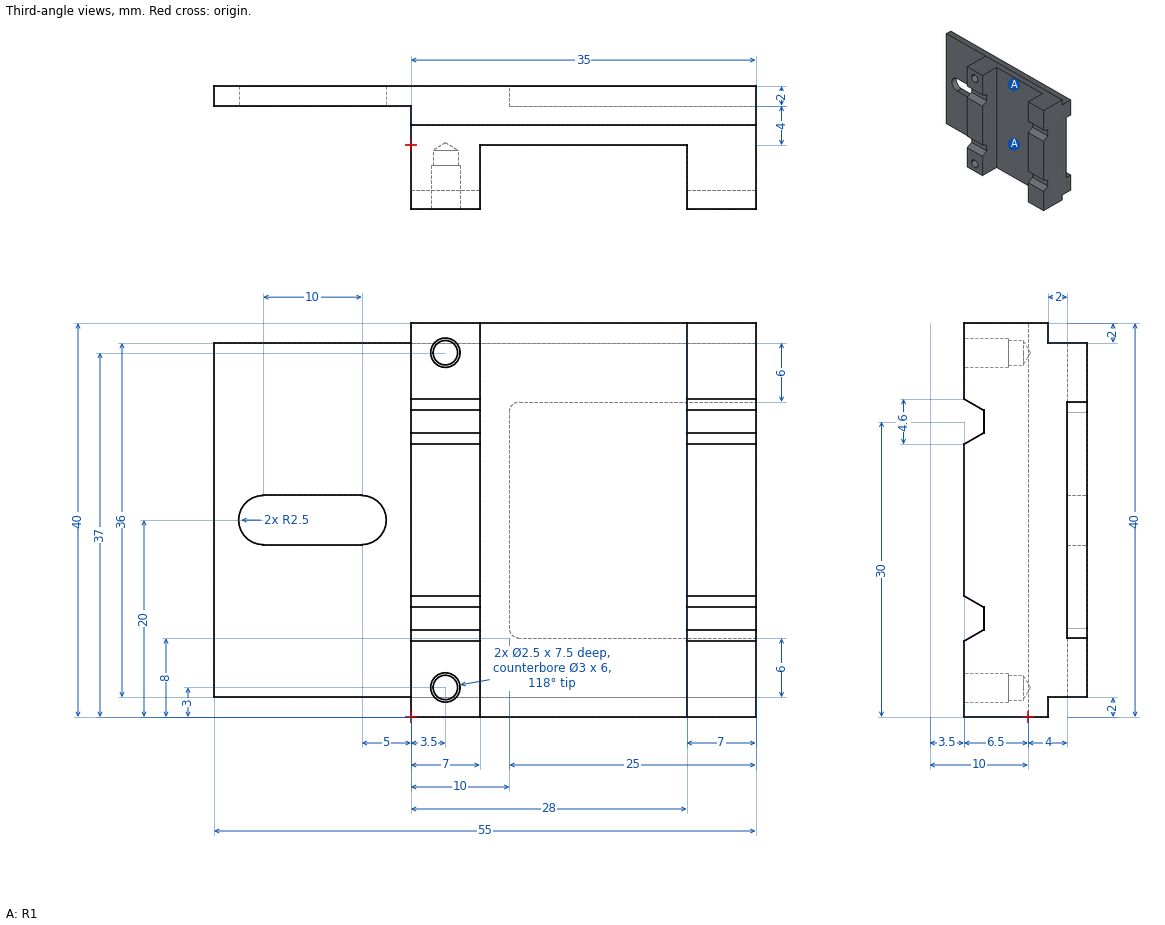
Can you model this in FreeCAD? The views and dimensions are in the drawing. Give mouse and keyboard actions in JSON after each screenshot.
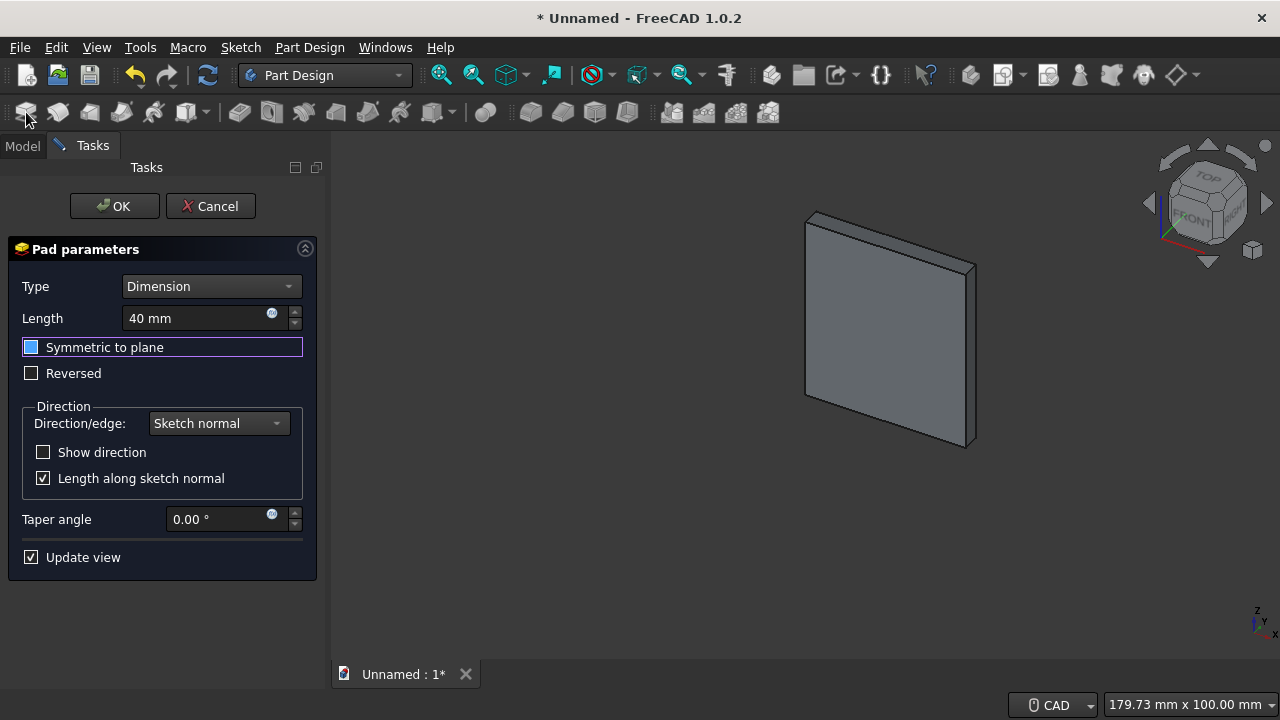
{"action": "left_click", "coordinate": [115, 206]}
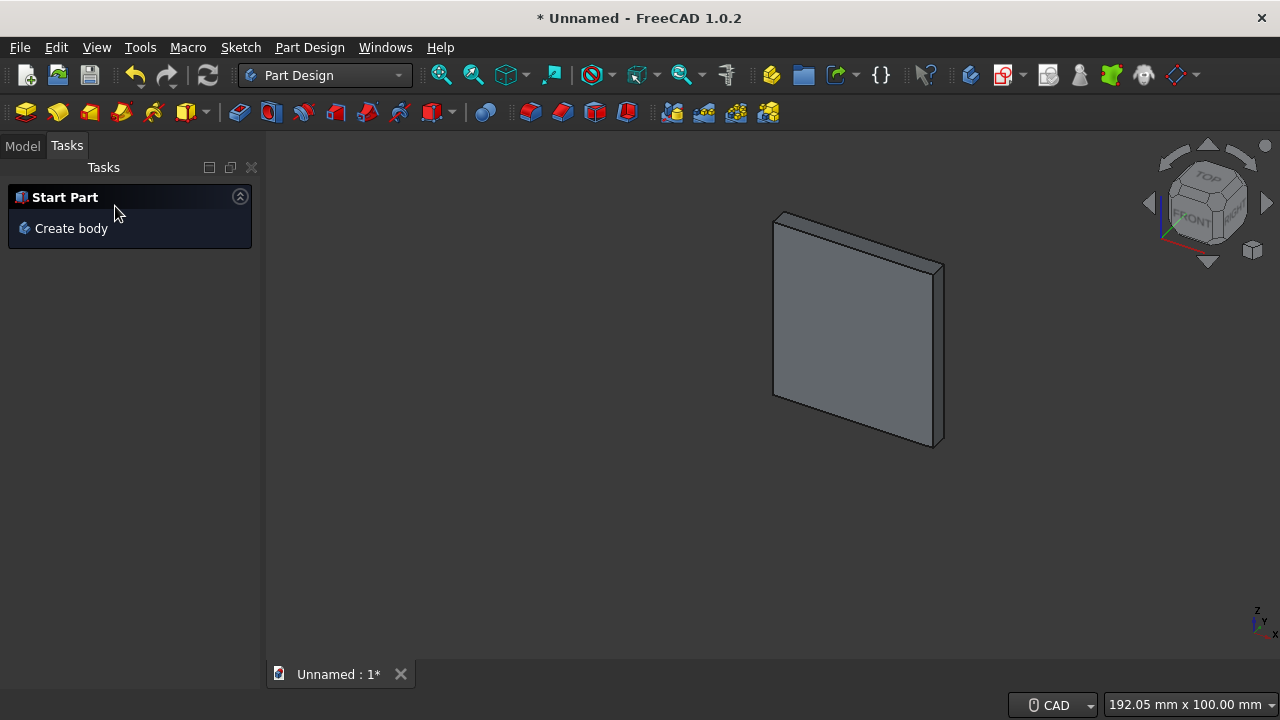
{"action": "left_click", "coordinate": [442, 76]}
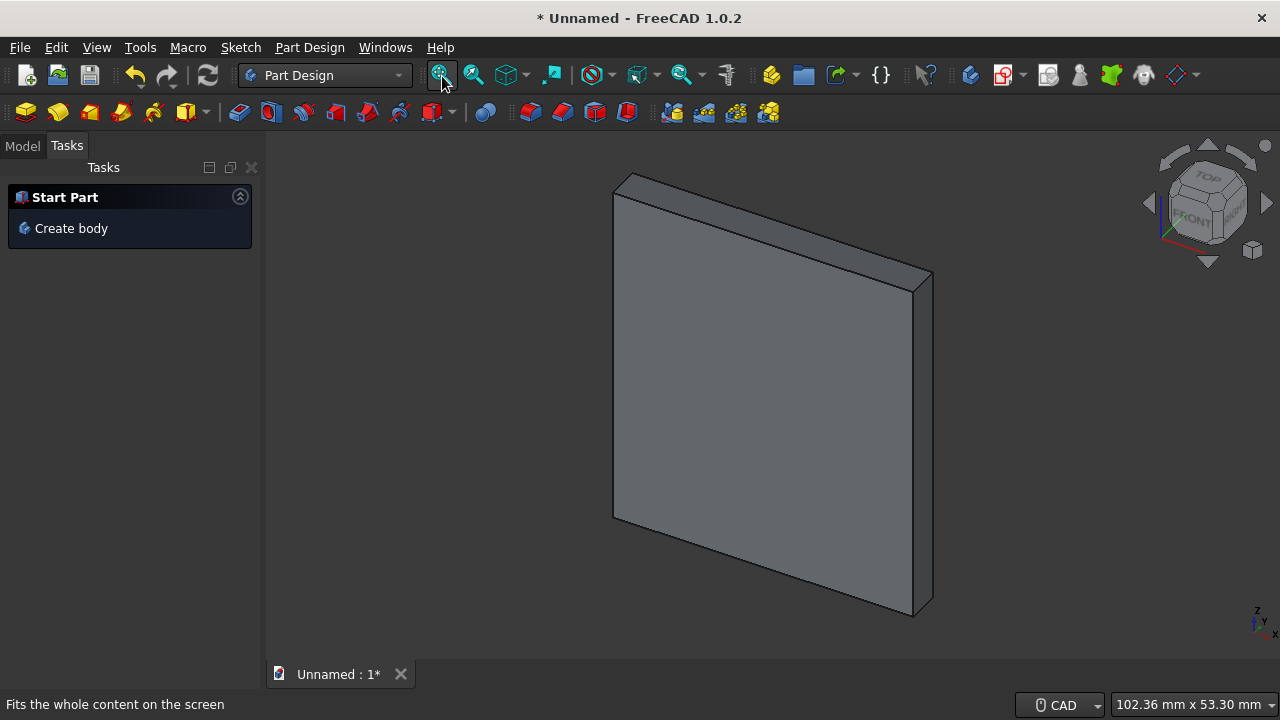
{"action": "key", "text": "4"}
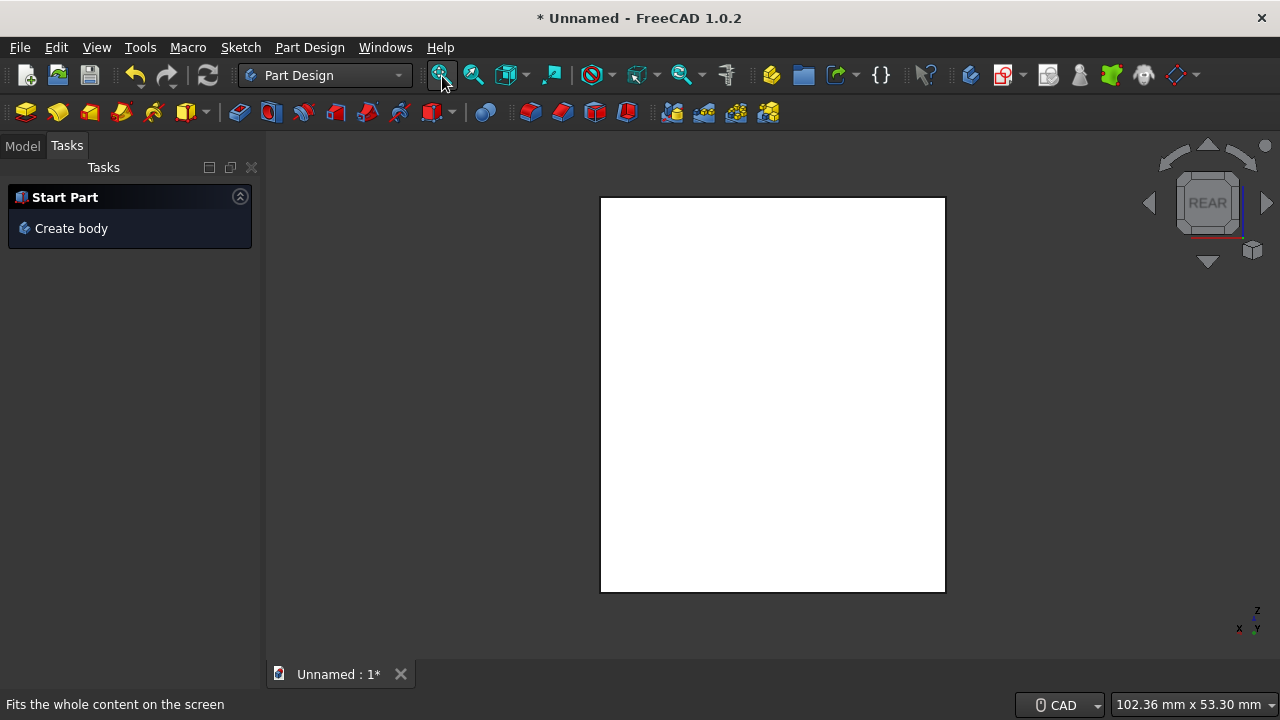
{"action": "left_click", "coordinate": [773, 394]}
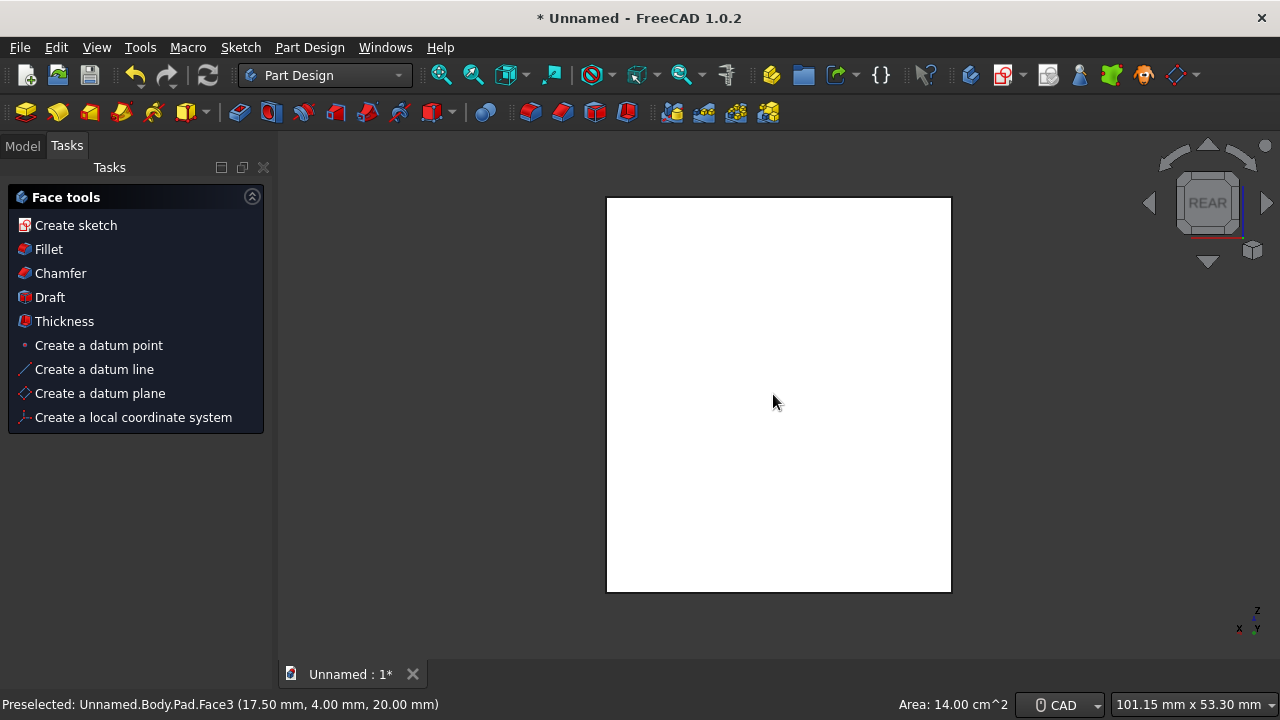
{"action": "left_click", "coordinate": [1004, 76]}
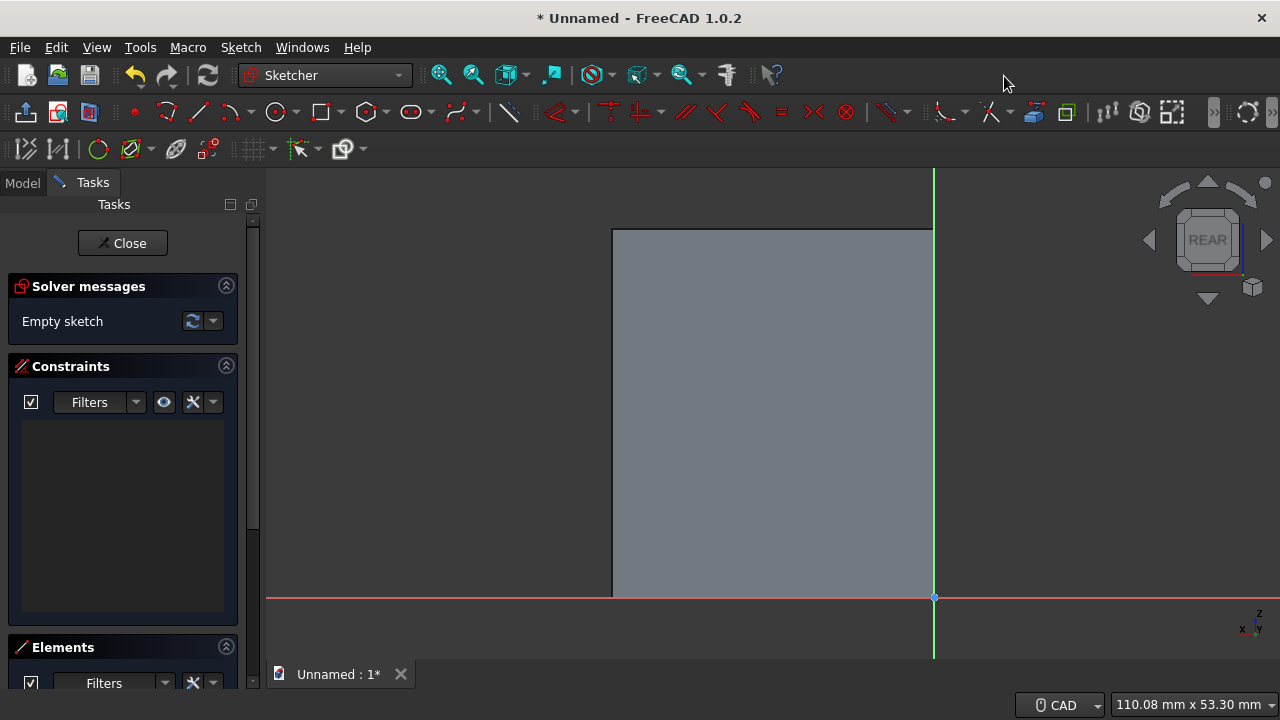
{"action": "left_click", "coordinate": [322, 112]}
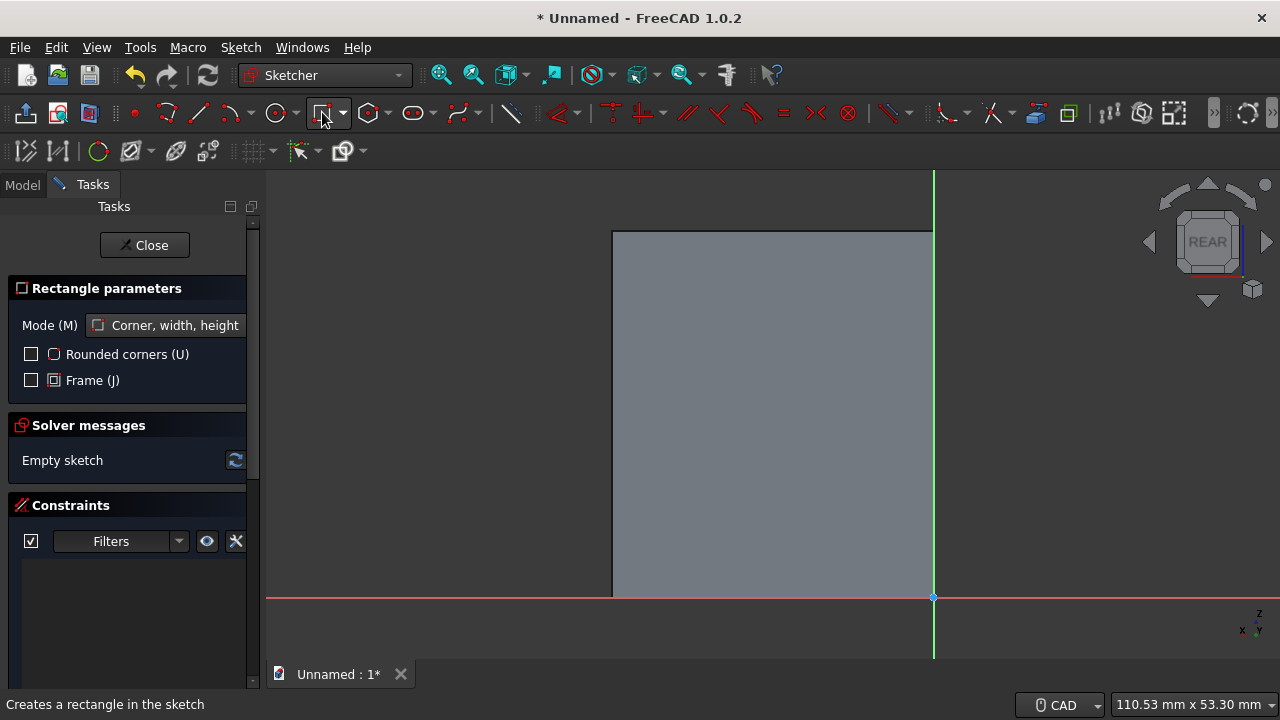
{"action": "left_click", "coordinate": [934, 598]}
{"action": "mouse_move", "coordinate": [869, 231]}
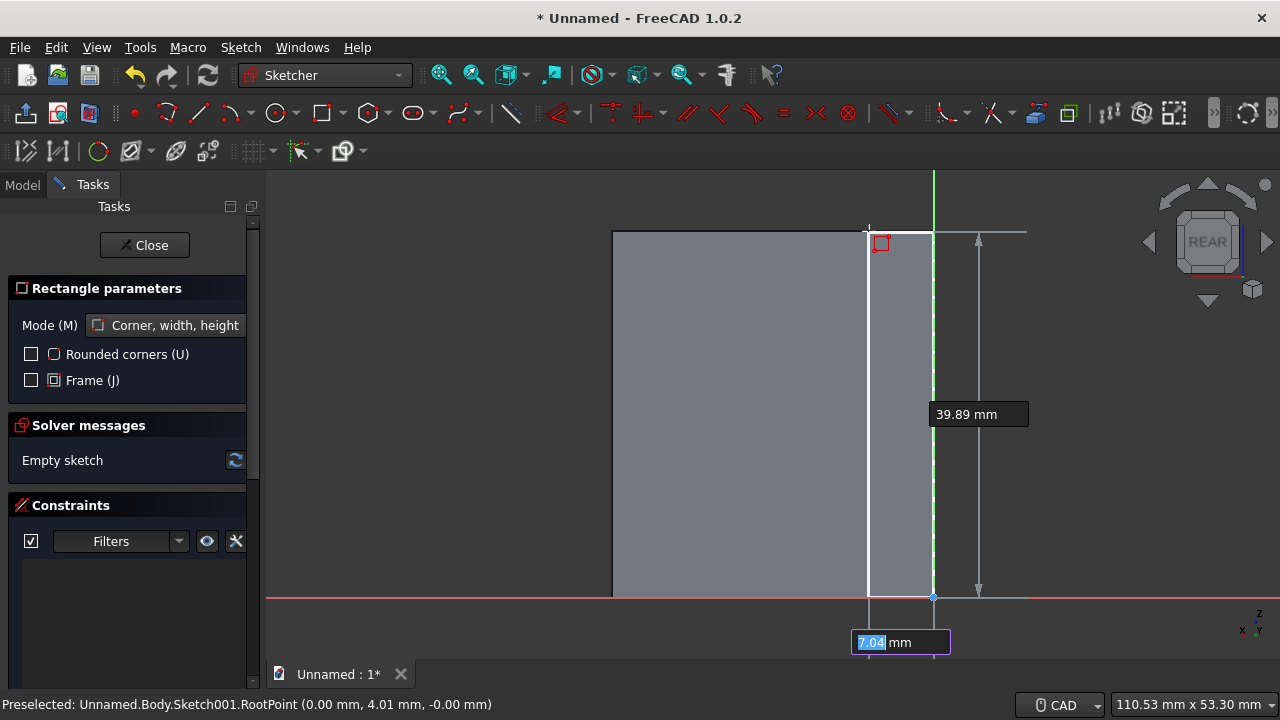
{"action": "type", "text": "7"}
{"action": "key", "text": "Tab"}
{"action": "type", "text": "40"}
{"action": "key", "text": "Return"}
{"action": "key", "text": "Escape"}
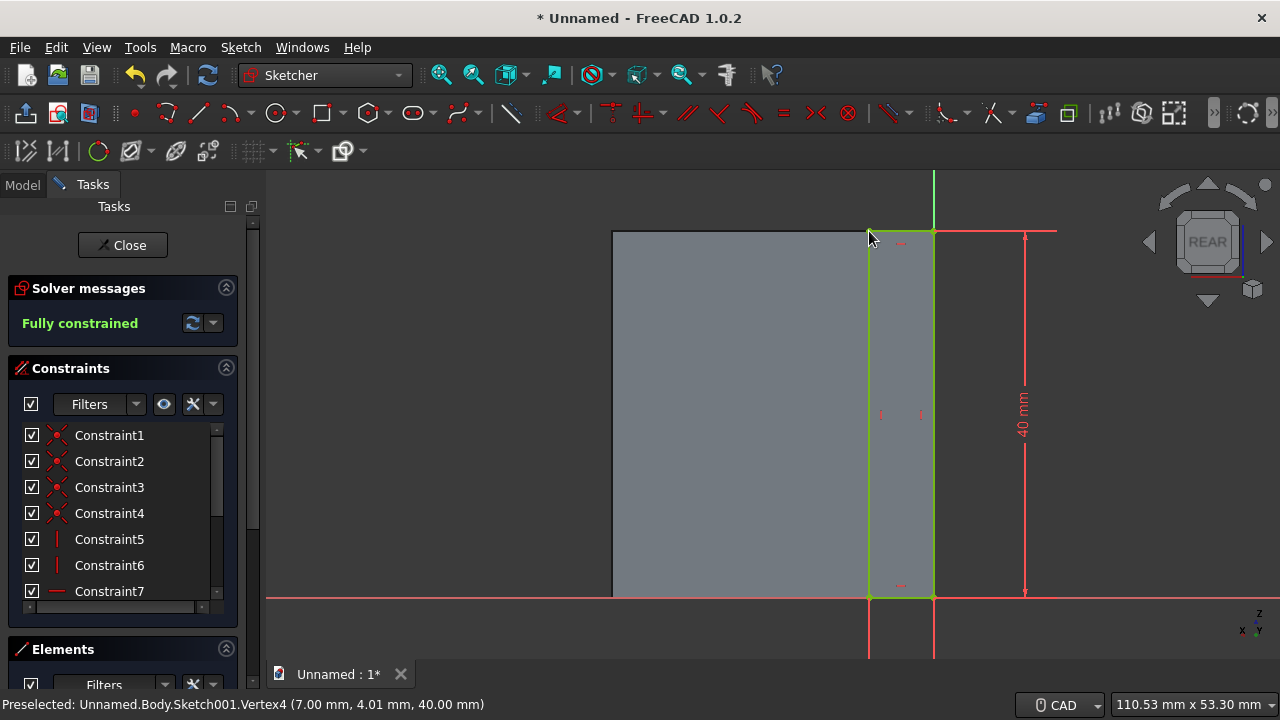
{"action": "left_click", "coordinate": [123, 245]}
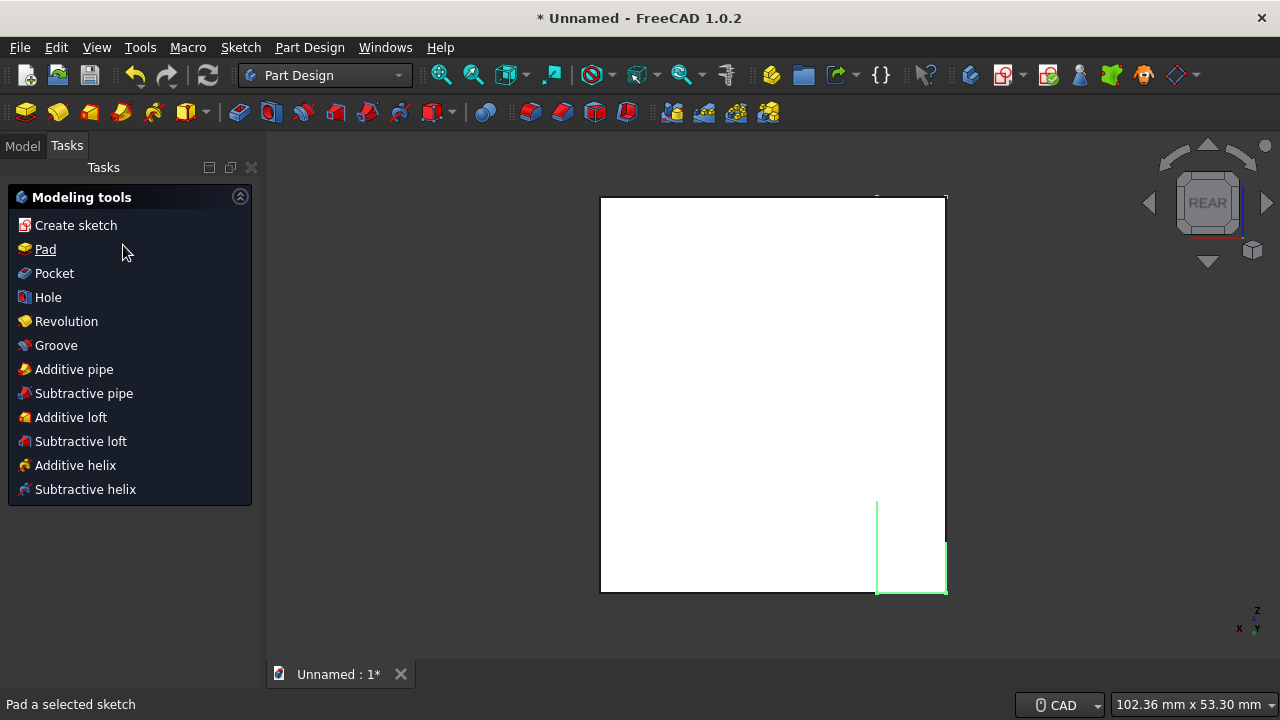
{"action": "left_click", "coordinate": [26, 112]}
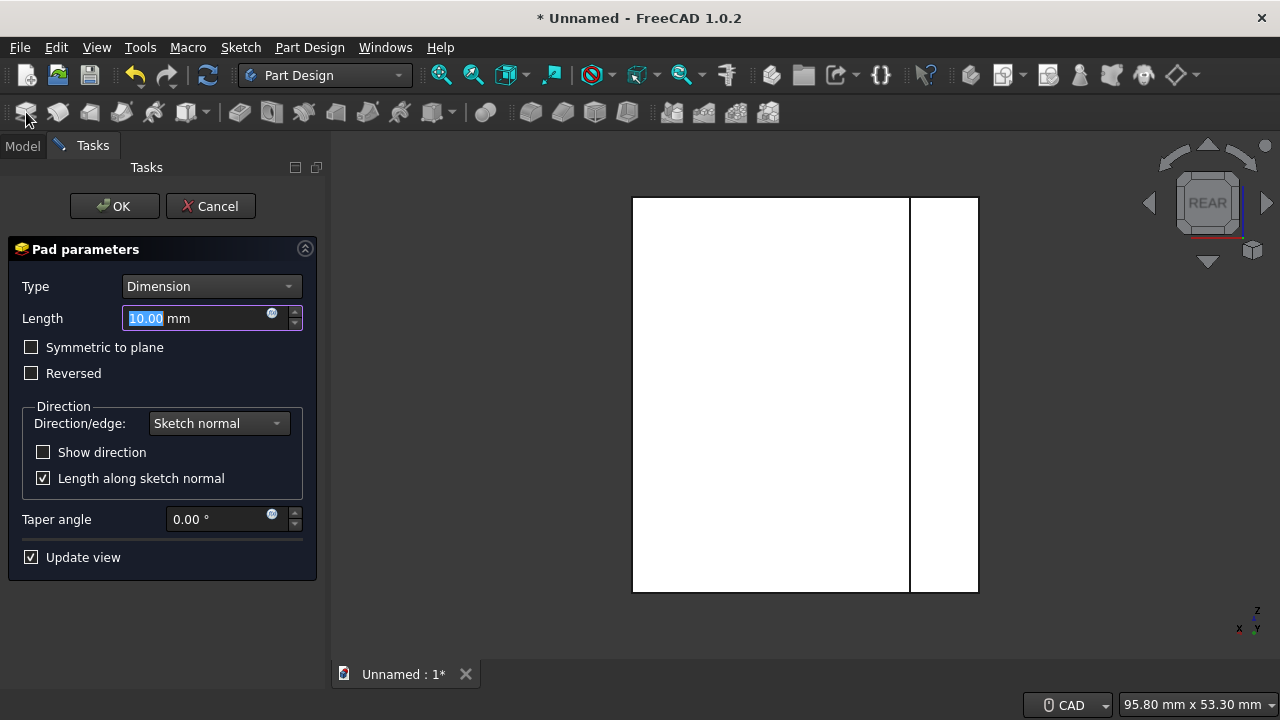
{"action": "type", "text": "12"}
{"action": "key", "text": "Tab"}